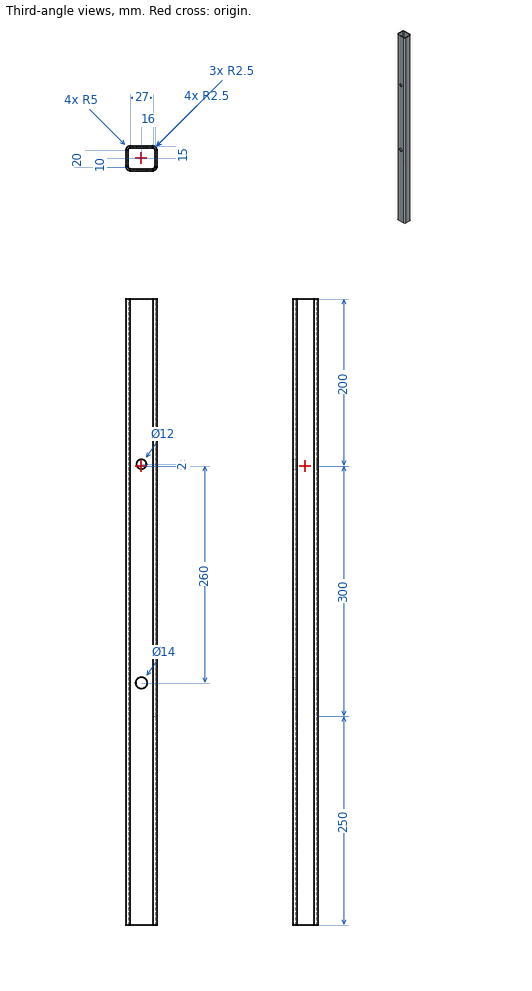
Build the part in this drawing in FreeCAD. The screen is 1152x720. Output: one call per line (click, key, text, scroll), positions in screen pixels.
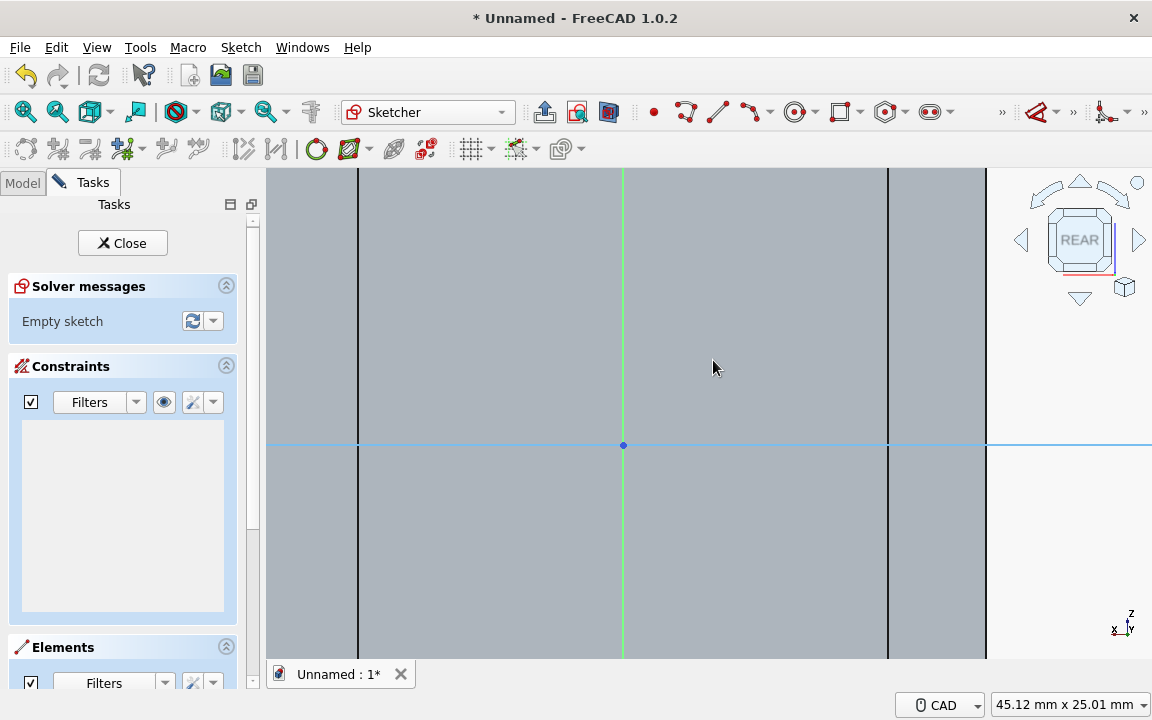
click(796, 112)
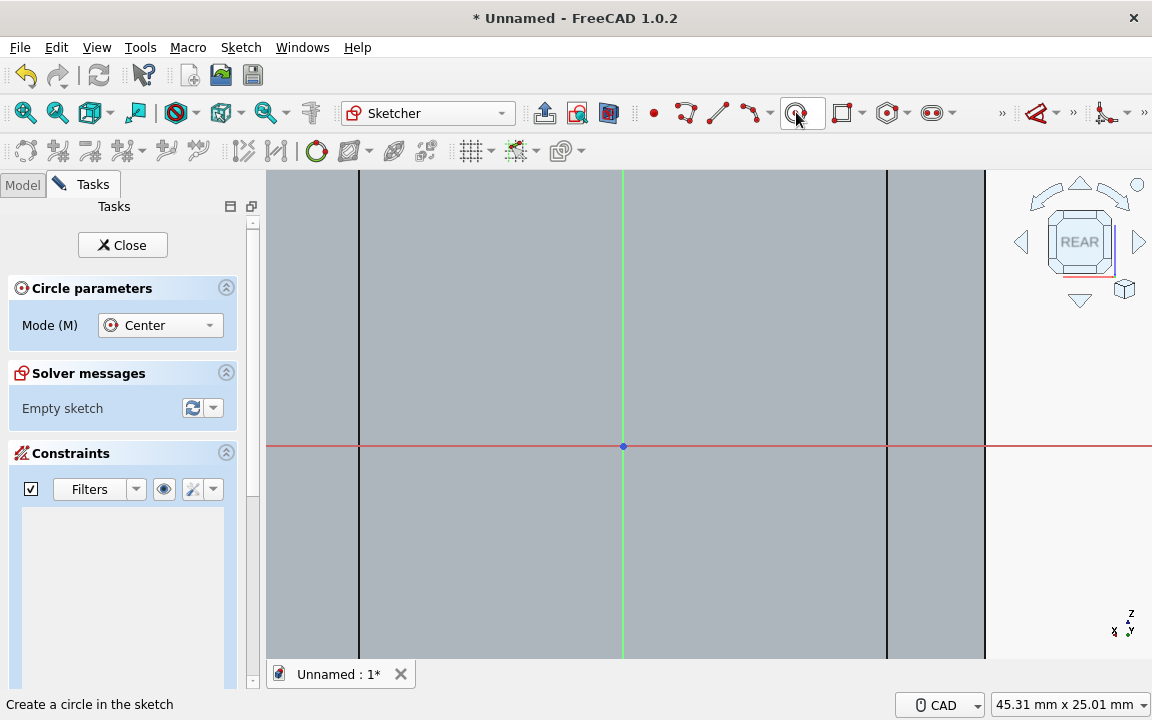
click(623, 407)
click(706, 324)
key(Escape)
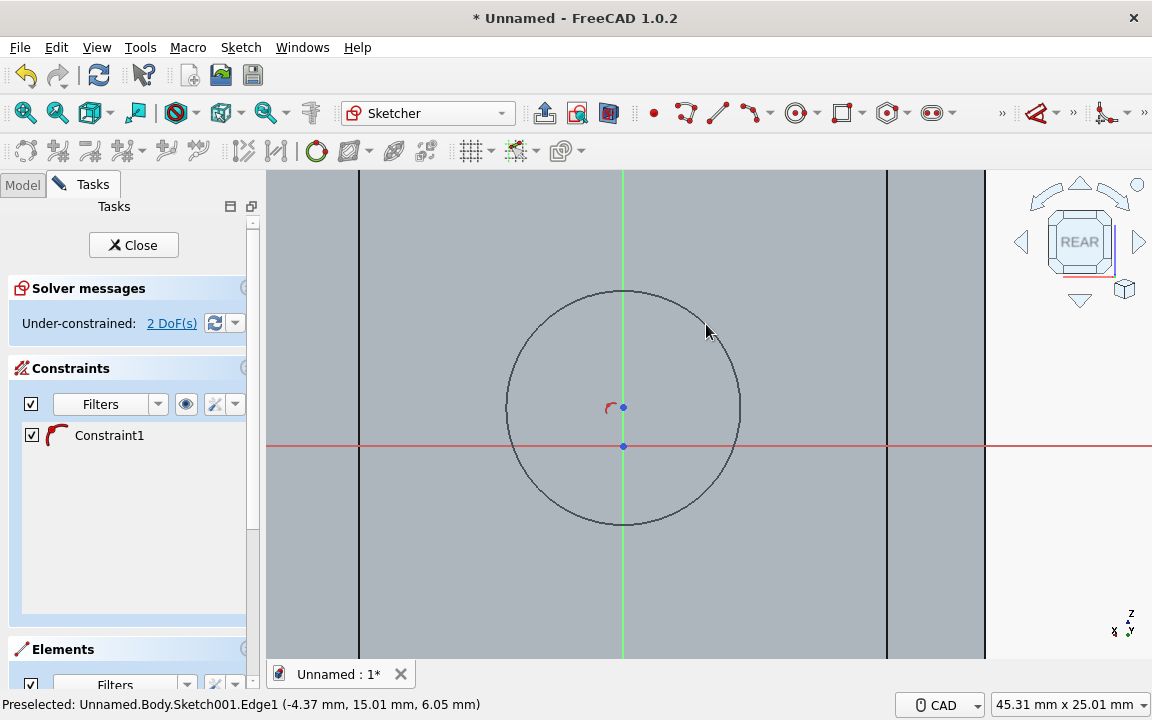
key(d)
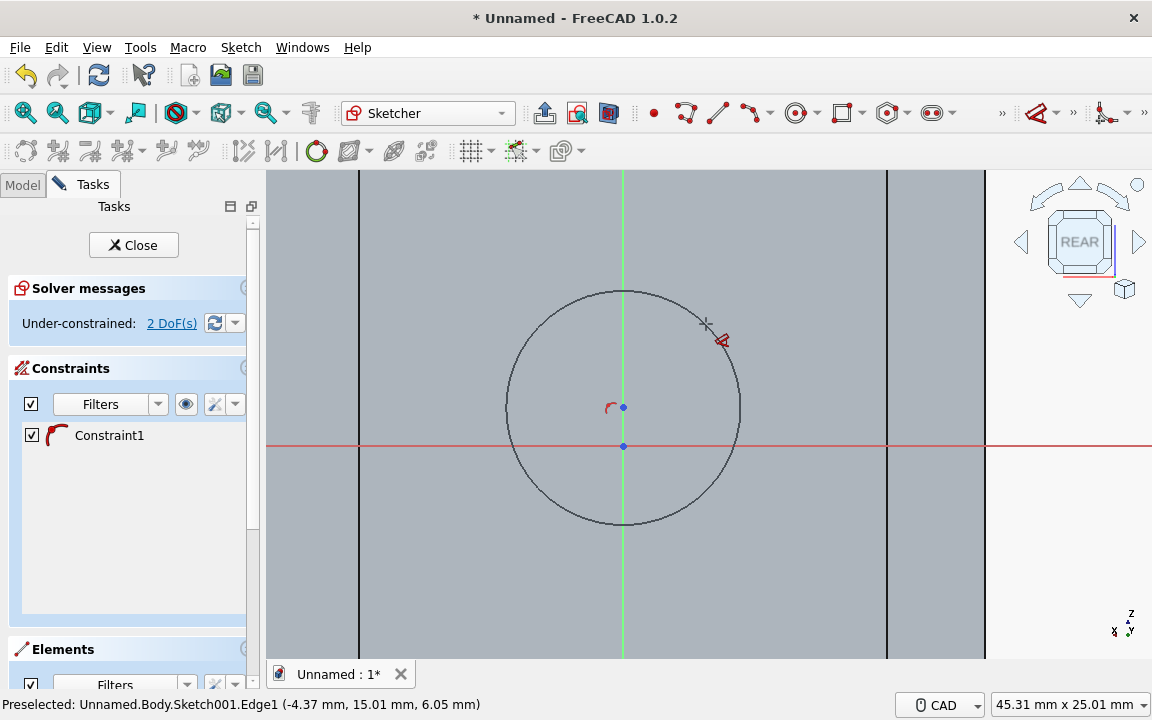
click(706, 325)
click(729, 302)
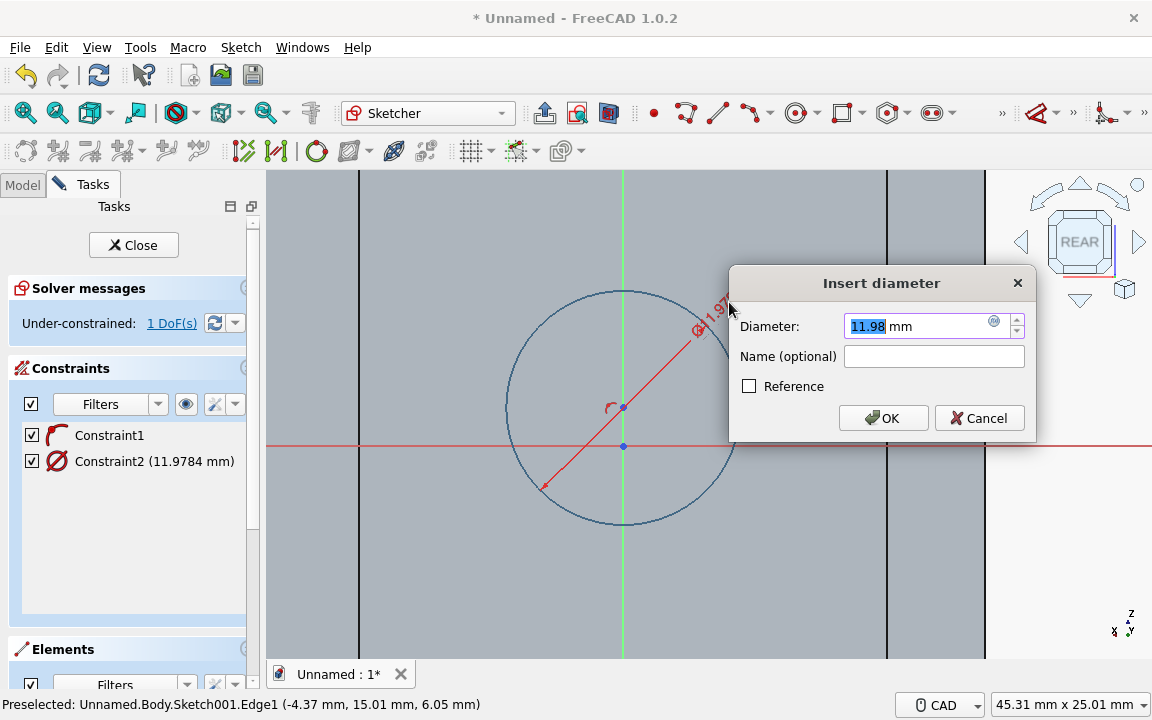
text(12)
key(Return)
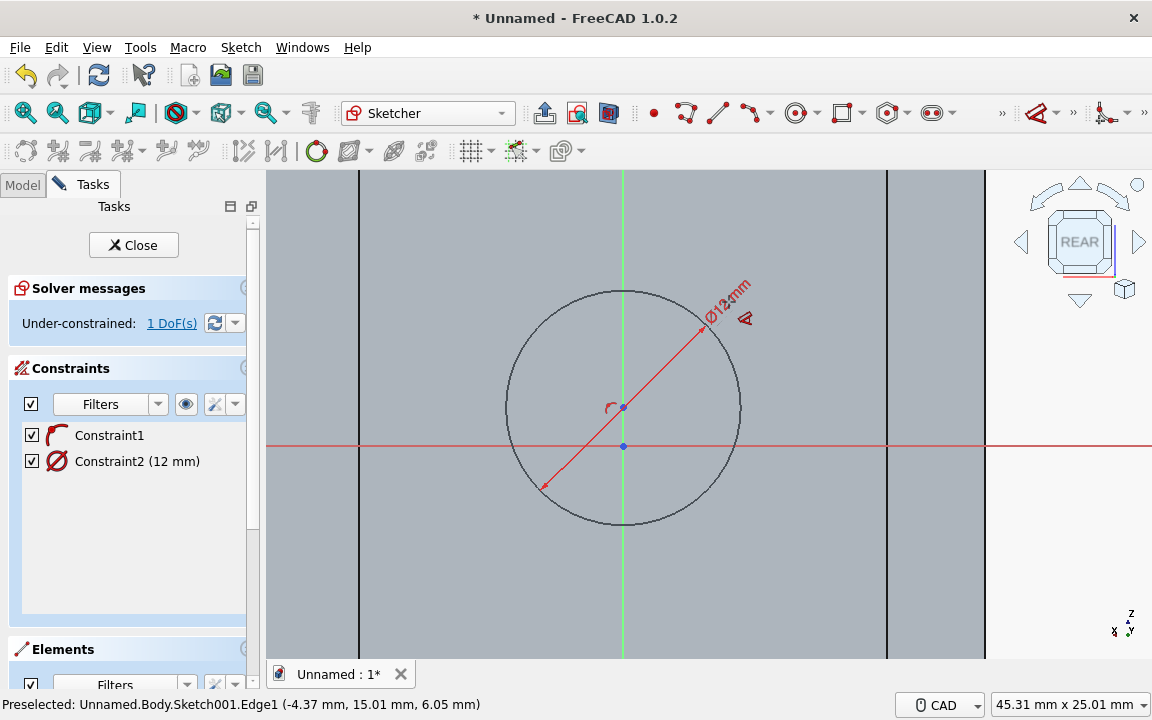
click(623, 408)
click(657, 427)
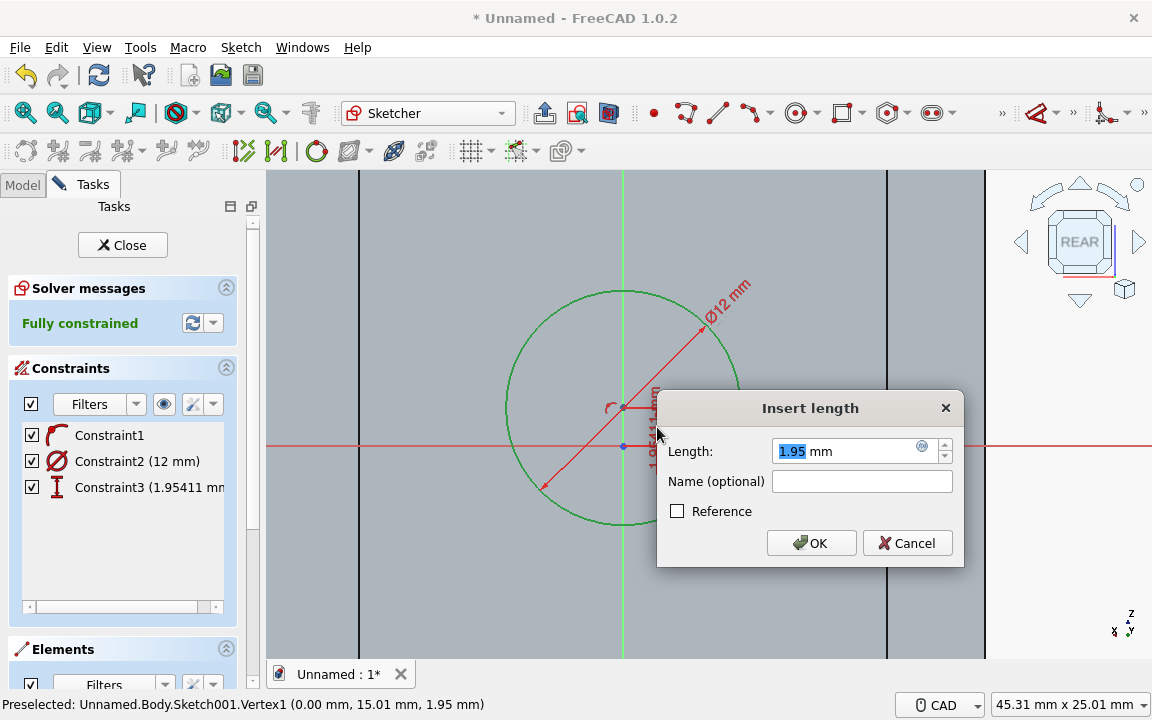
text(2)
key(Return)
key(Escape)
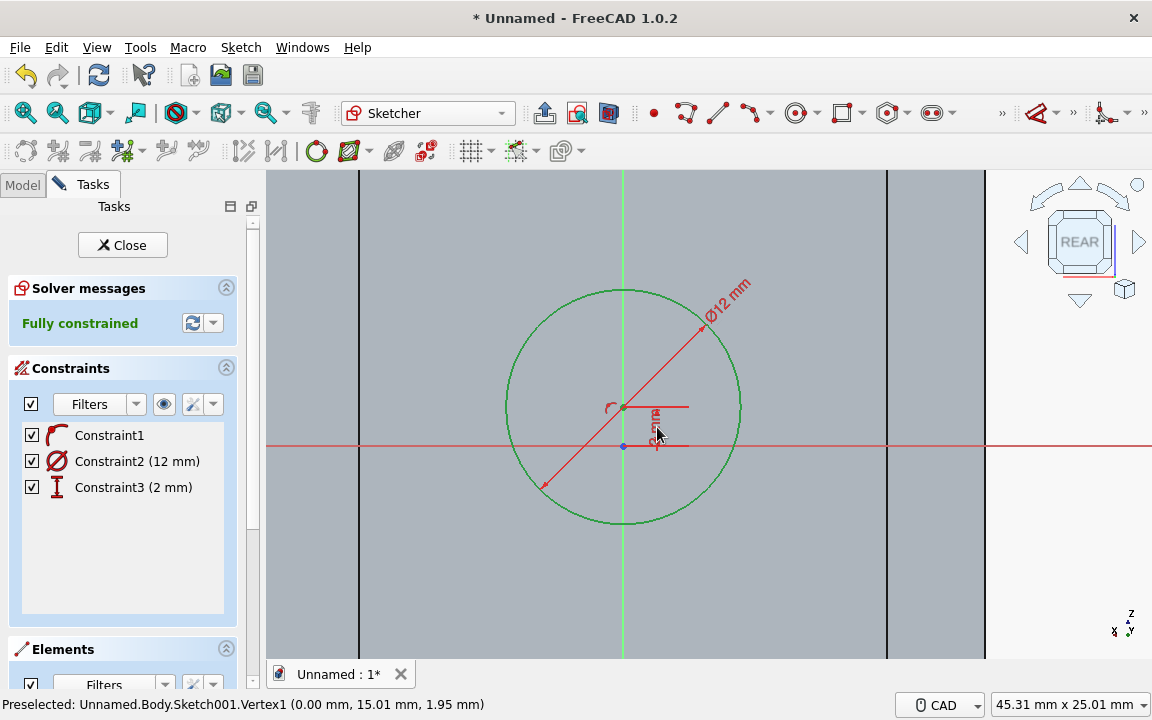
click(123, 245)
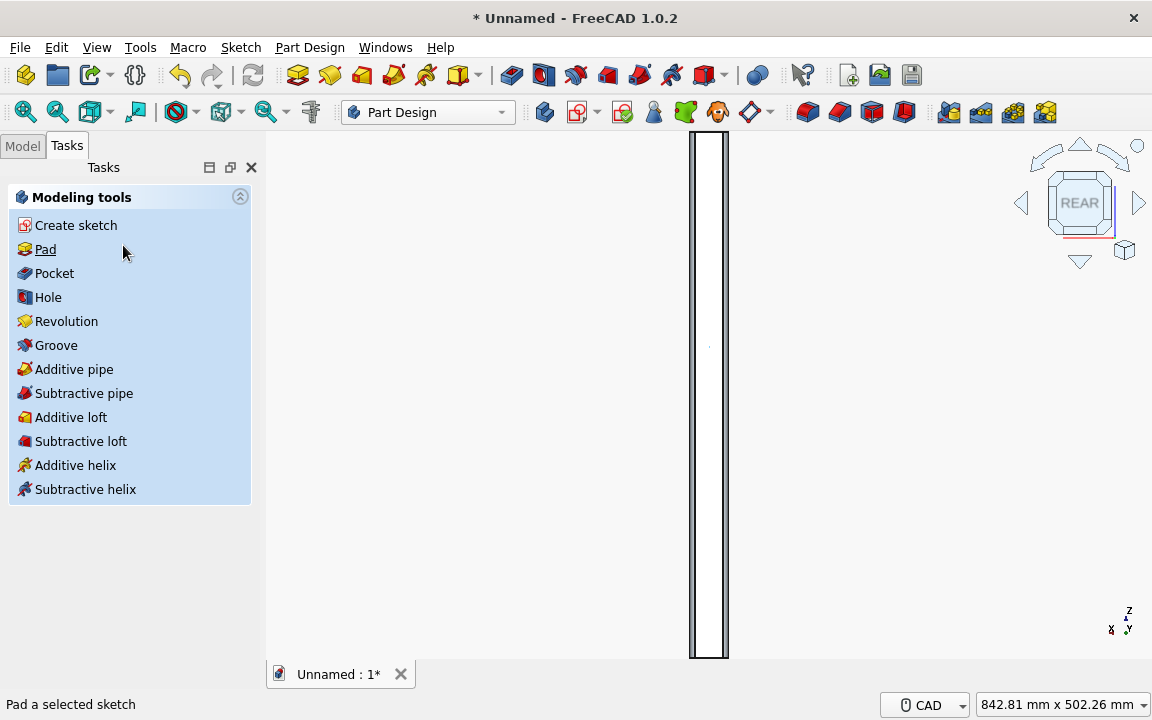
click(512, 76)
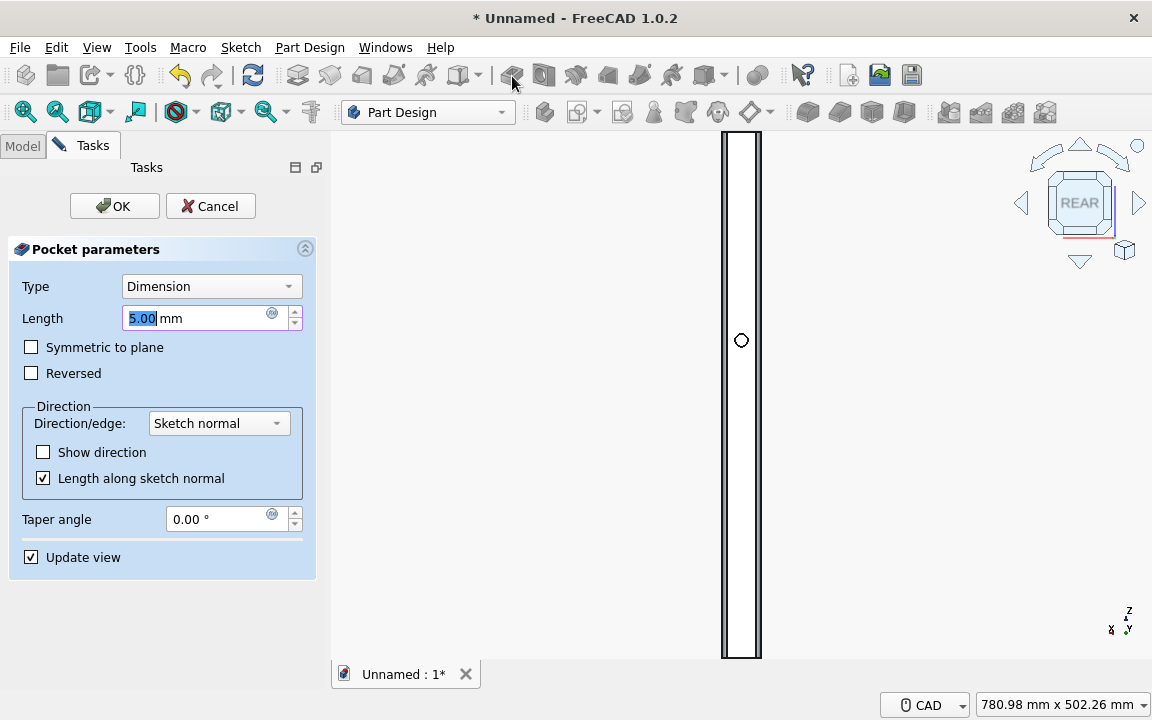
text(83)
key(Tab)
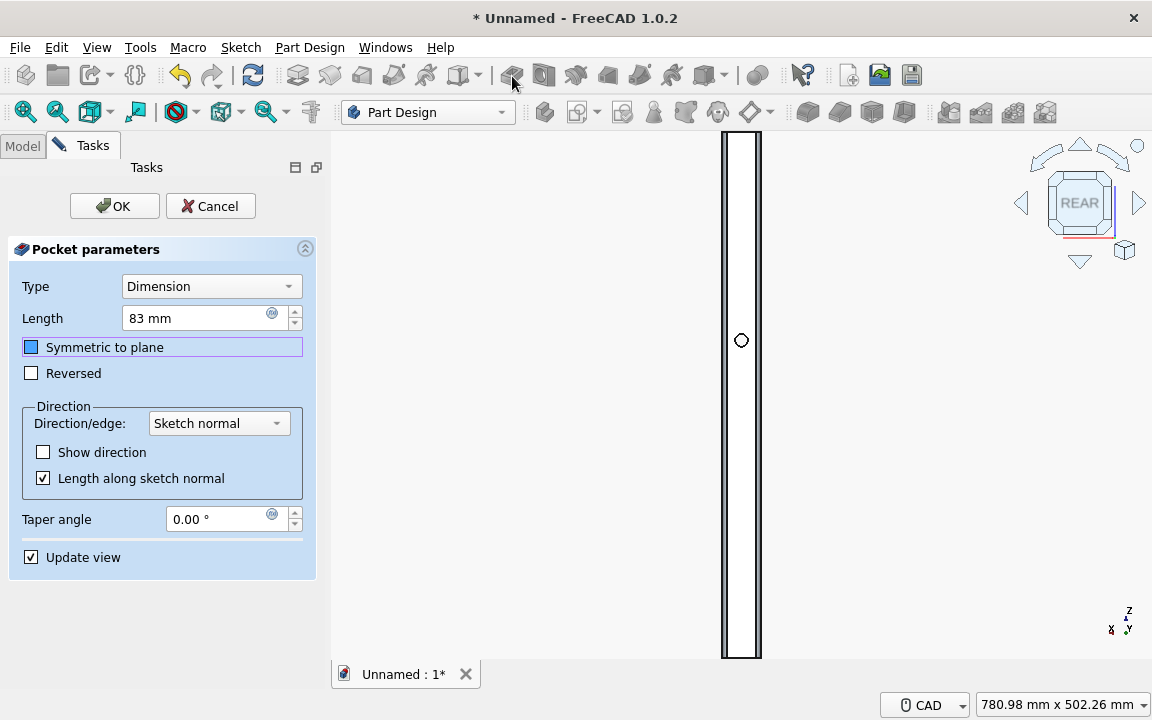
click(115, 206)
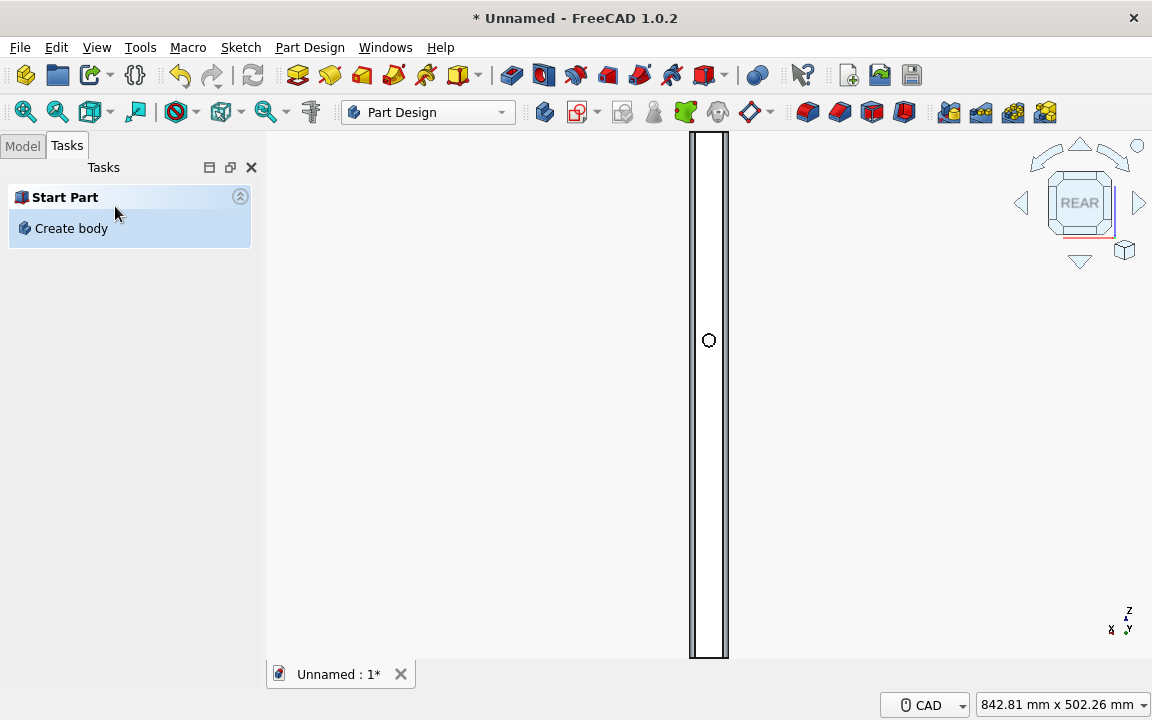
click(709, 169)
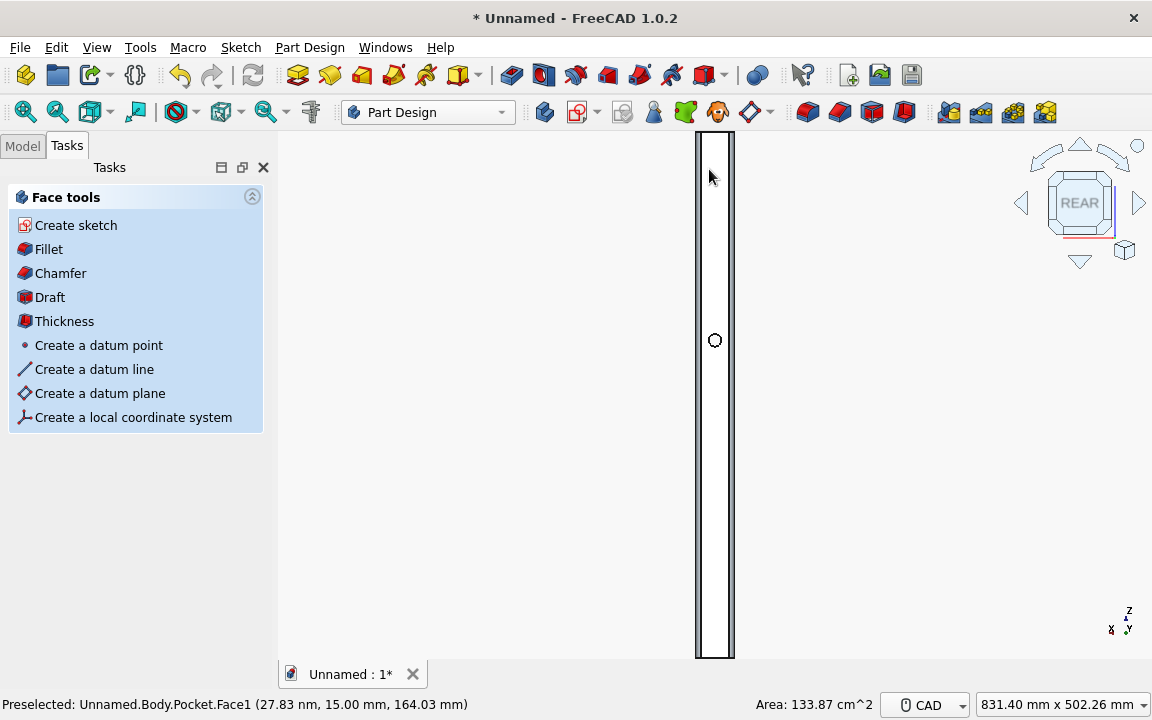
click(578, 112)